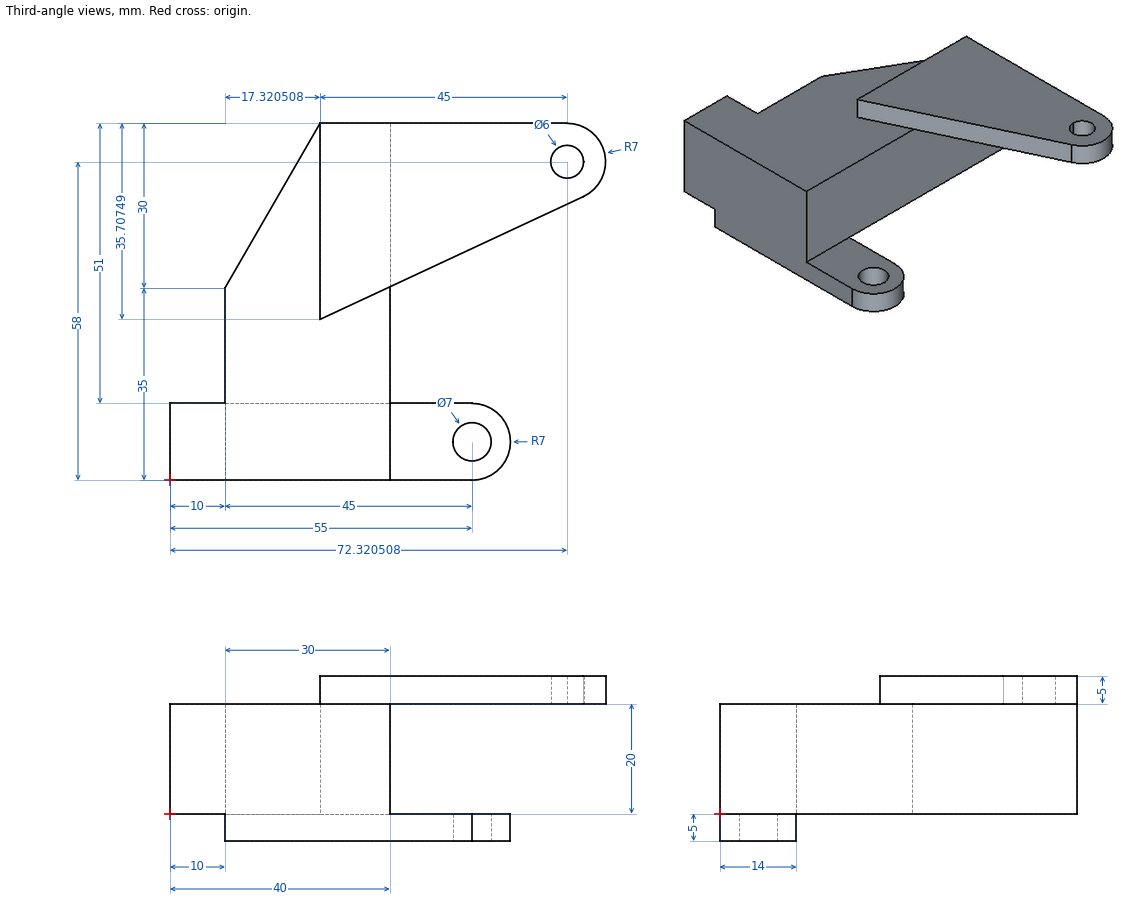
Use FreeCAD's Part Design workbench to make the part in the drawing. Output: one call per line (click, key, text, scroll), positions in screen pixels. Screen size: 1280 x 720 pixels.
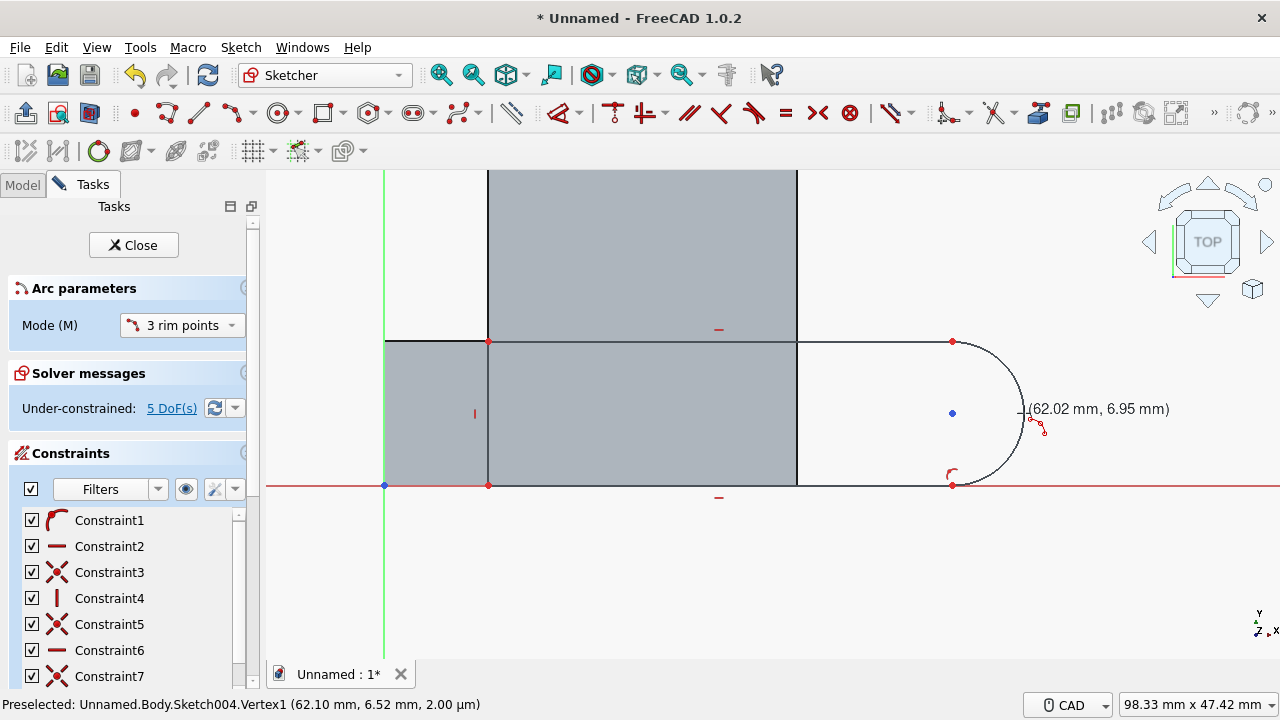
click(278, 114)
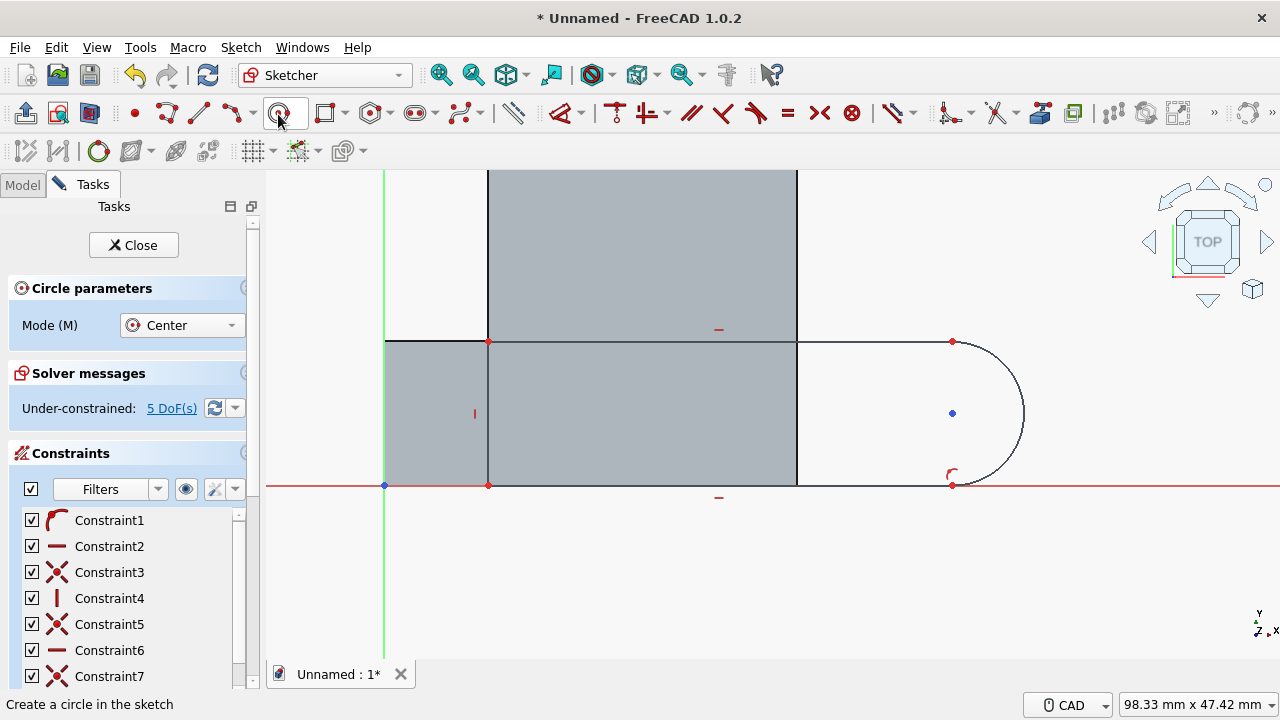
click(952, 413)
click(977, 388)
key(Escape)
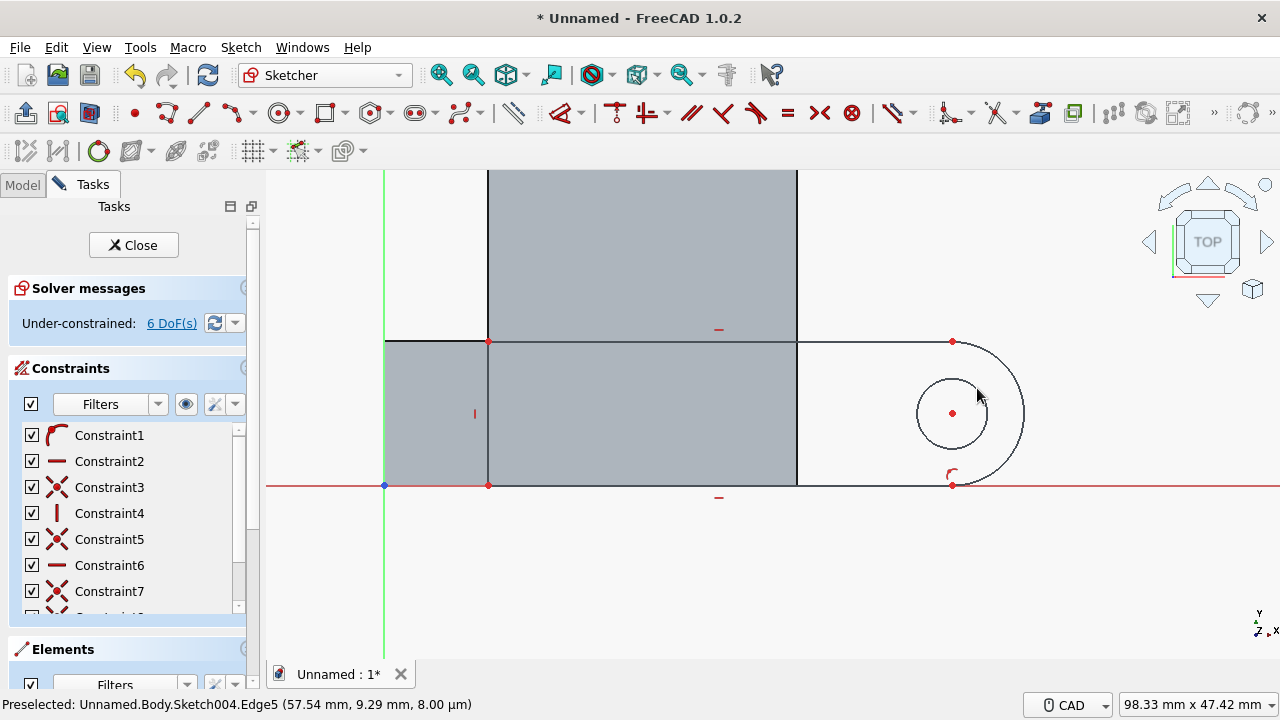
click(813, 486)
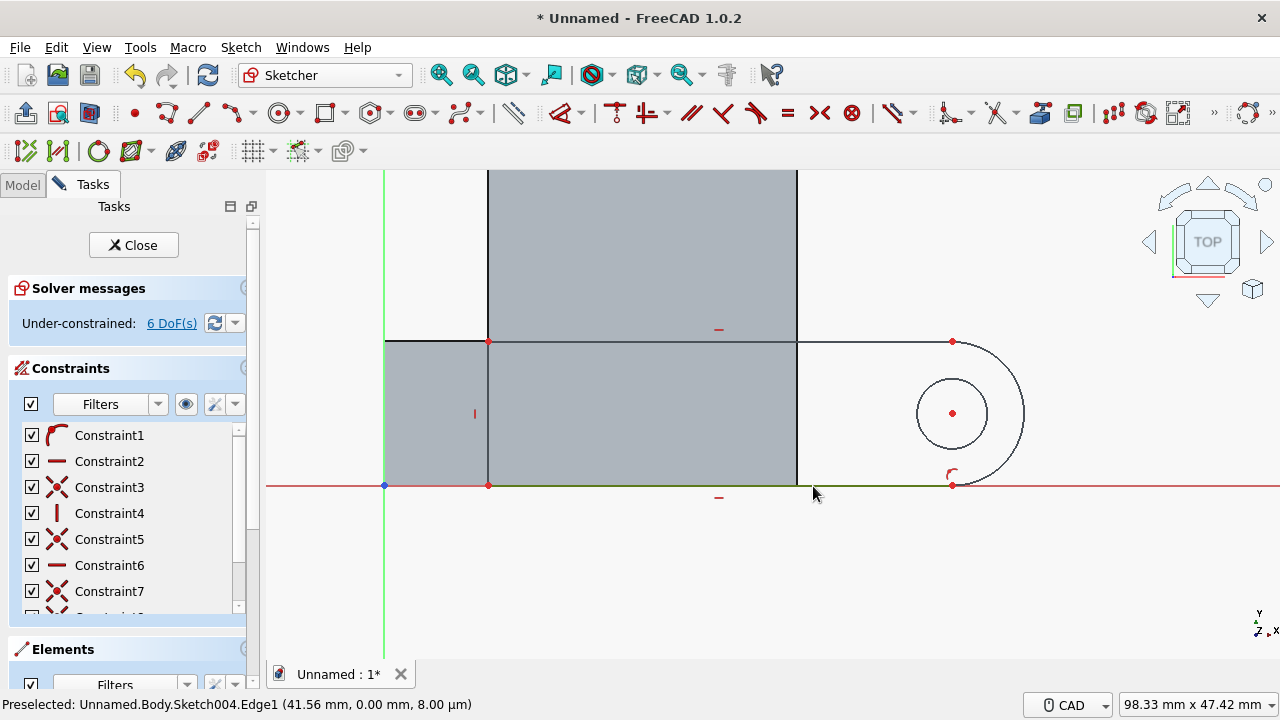
click(1010, 456)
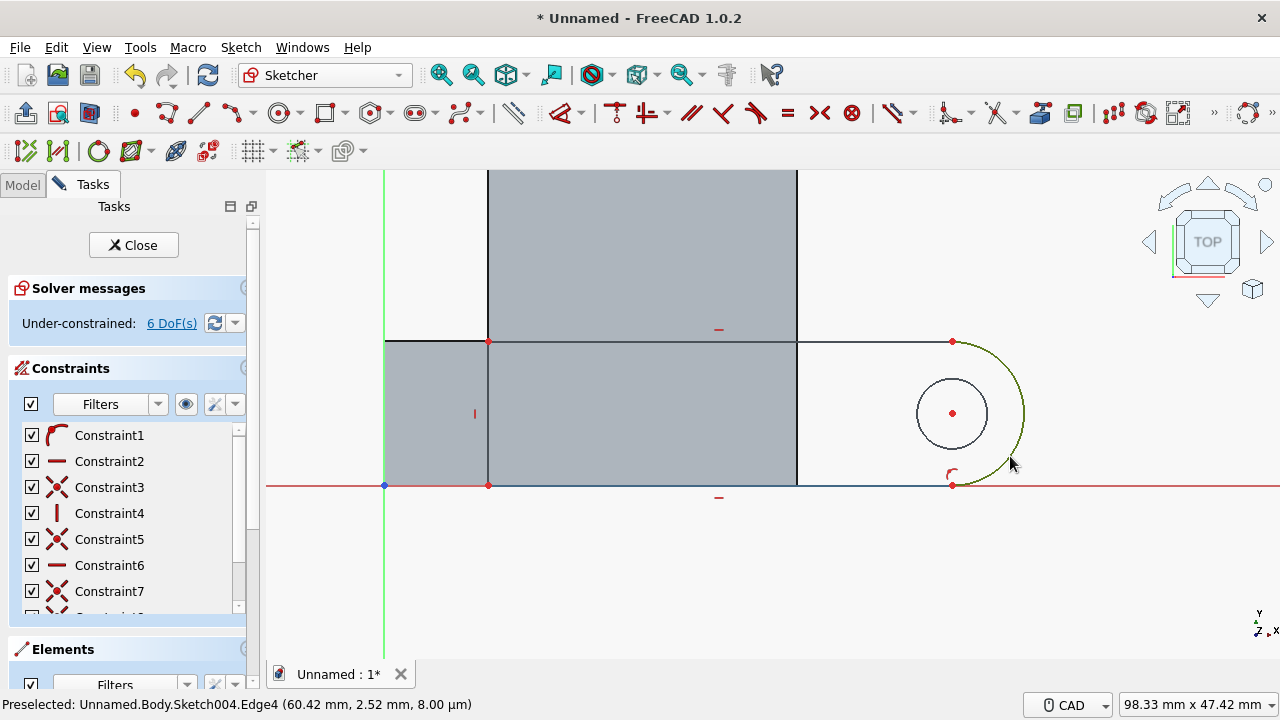
key(t)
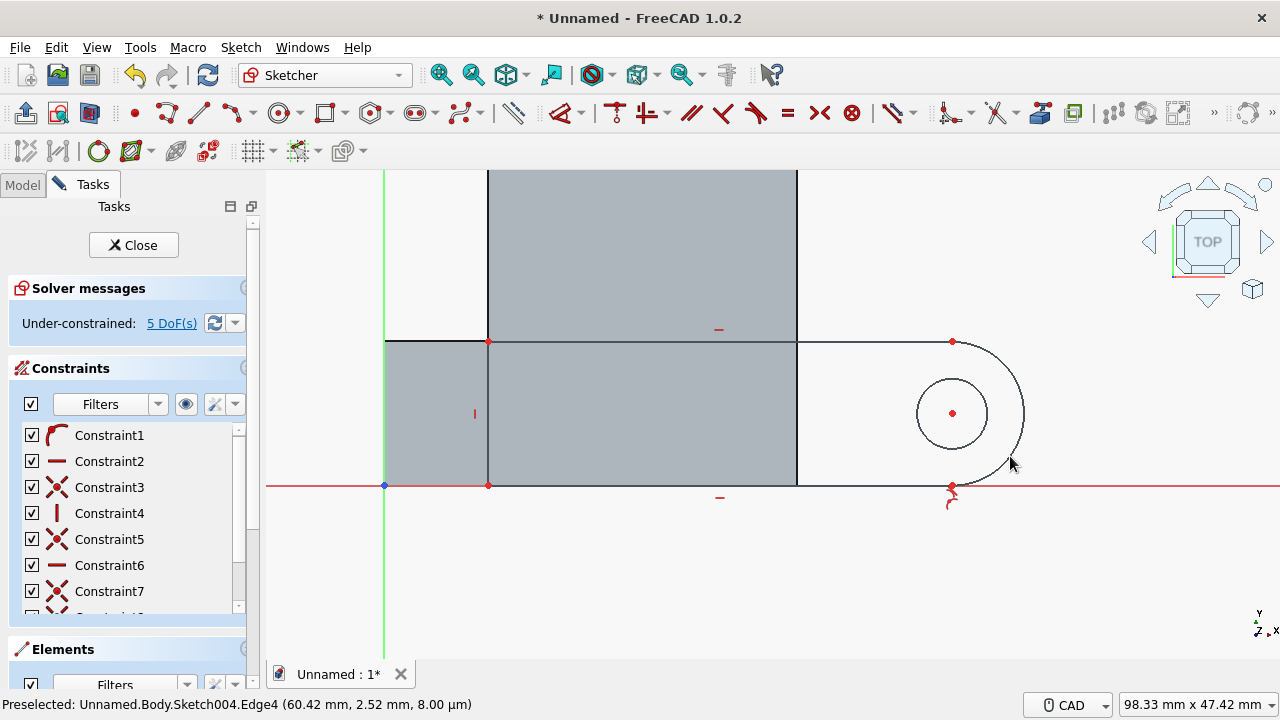
click(627, 342)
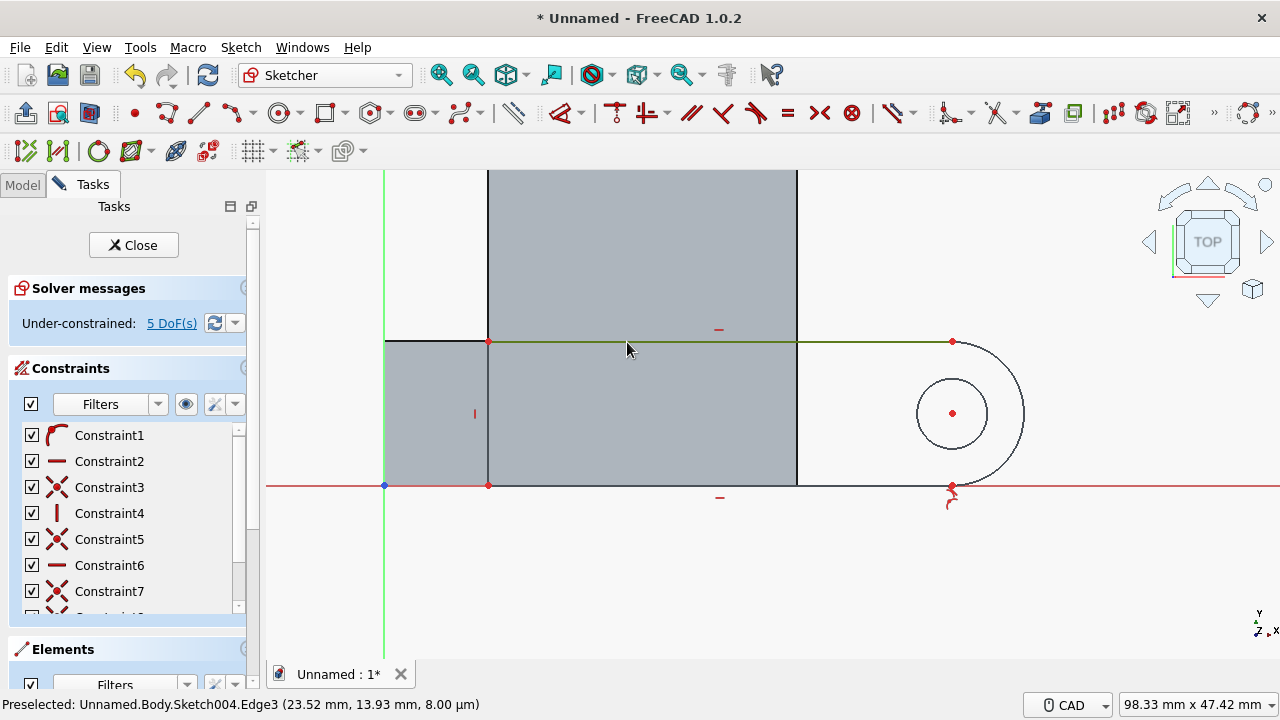
click(1010, 456)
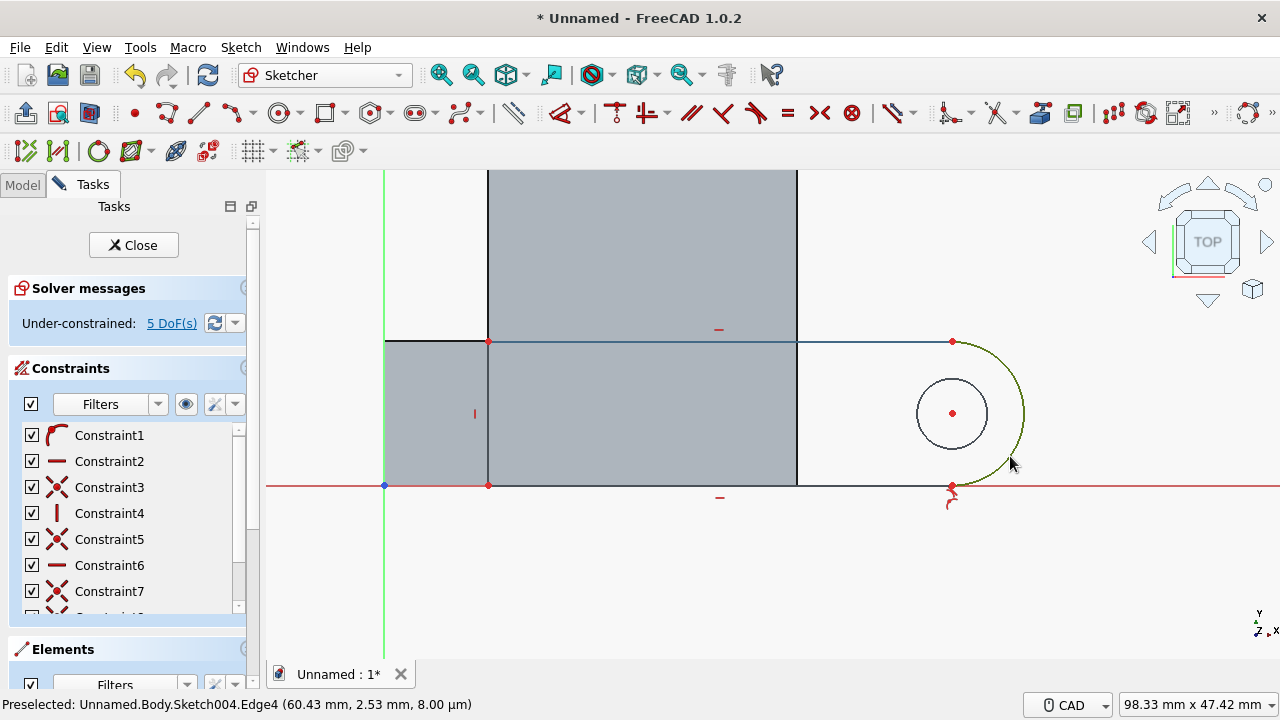
click(756, 114)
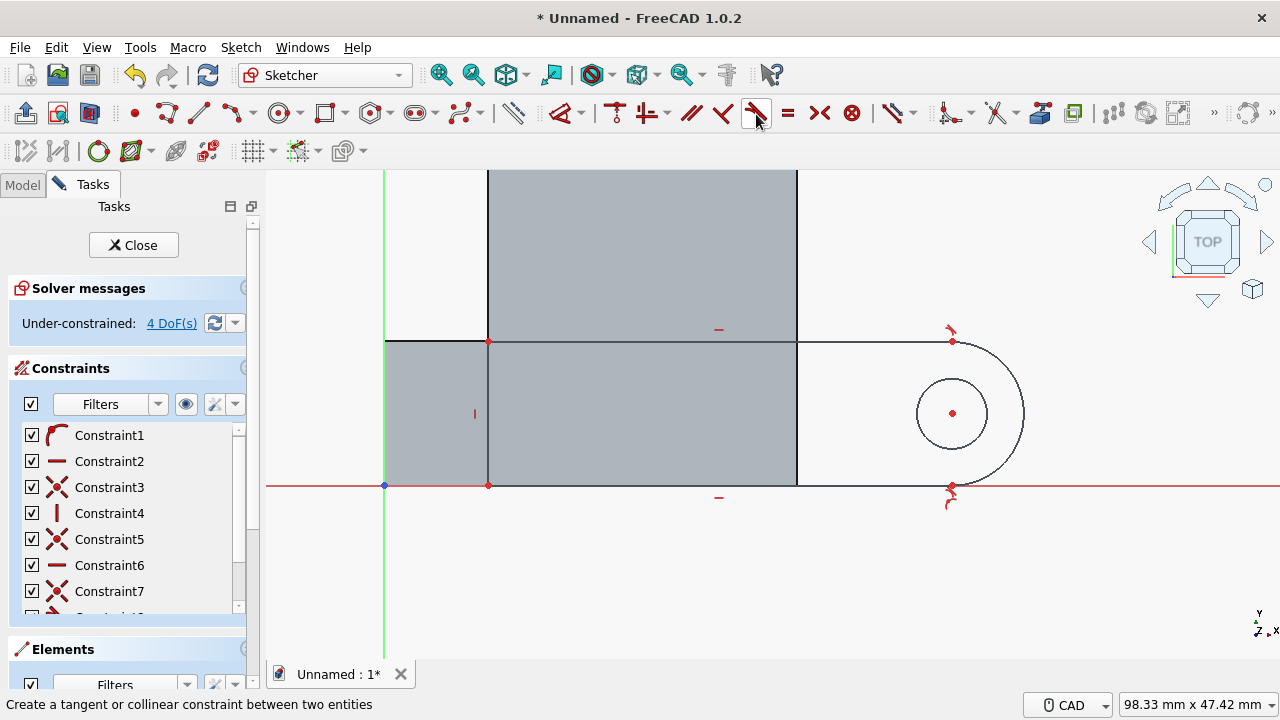
click(560, 114)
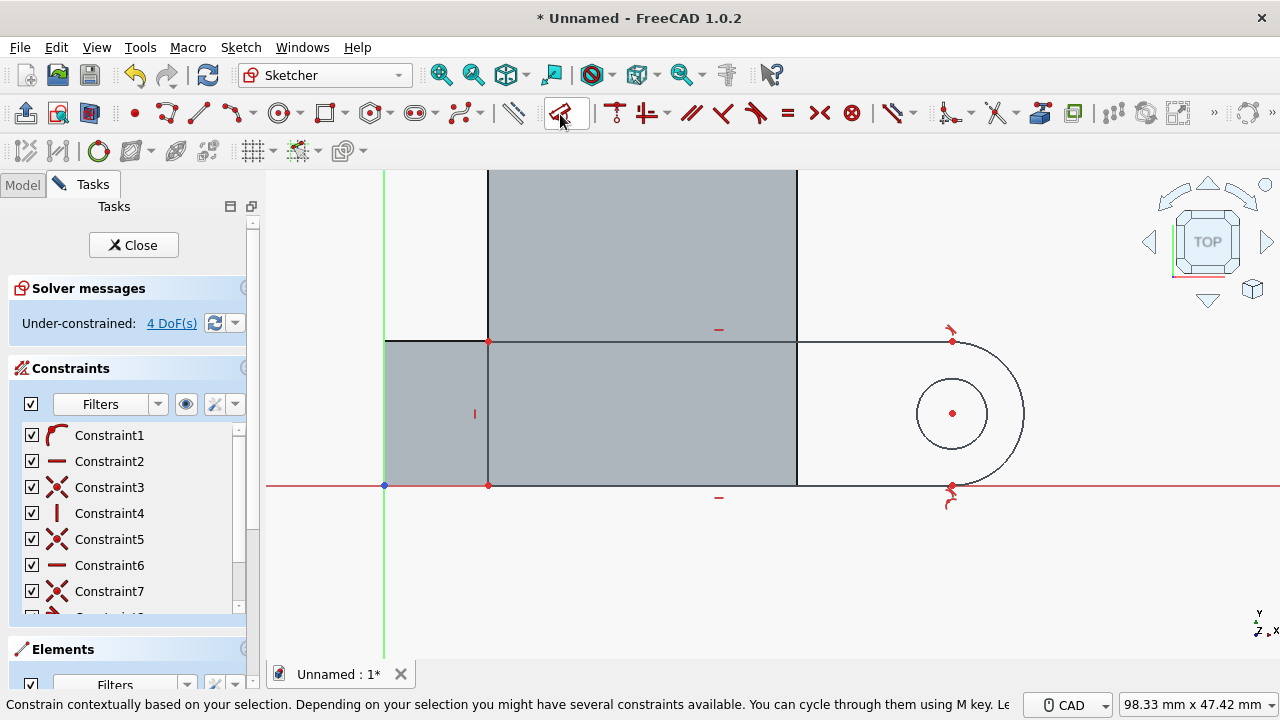
click(1010, 456)
click(996, 508)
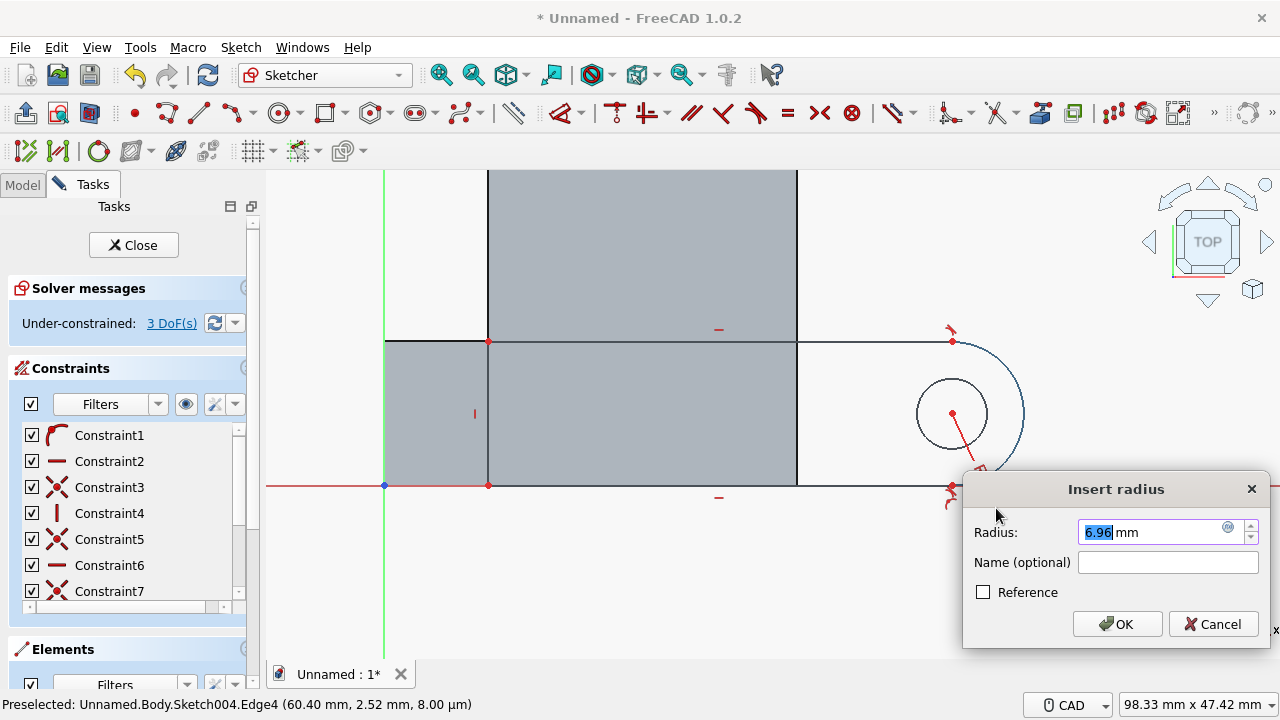
text(7)
key(Return)